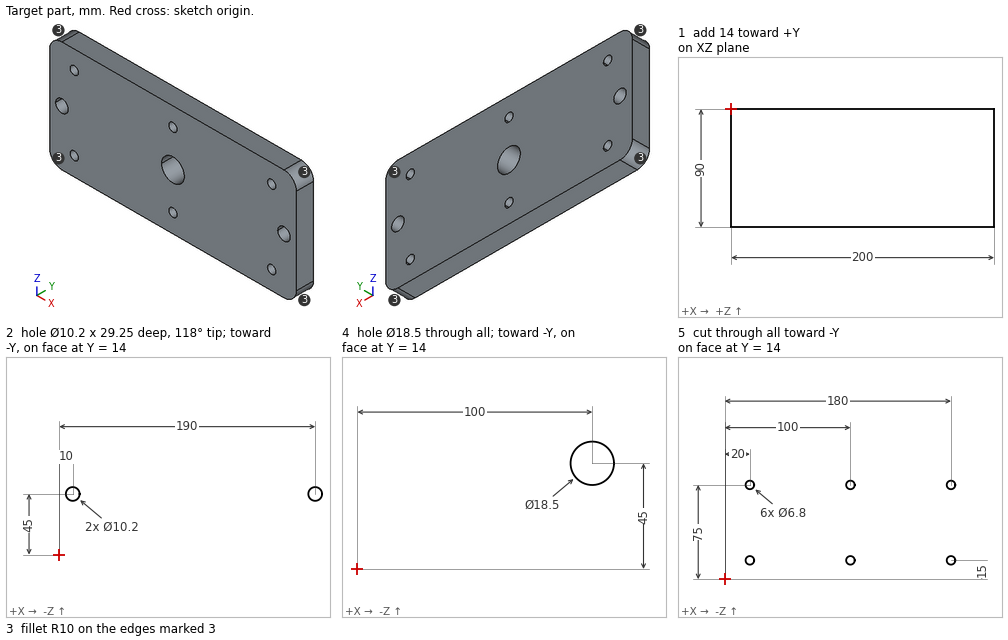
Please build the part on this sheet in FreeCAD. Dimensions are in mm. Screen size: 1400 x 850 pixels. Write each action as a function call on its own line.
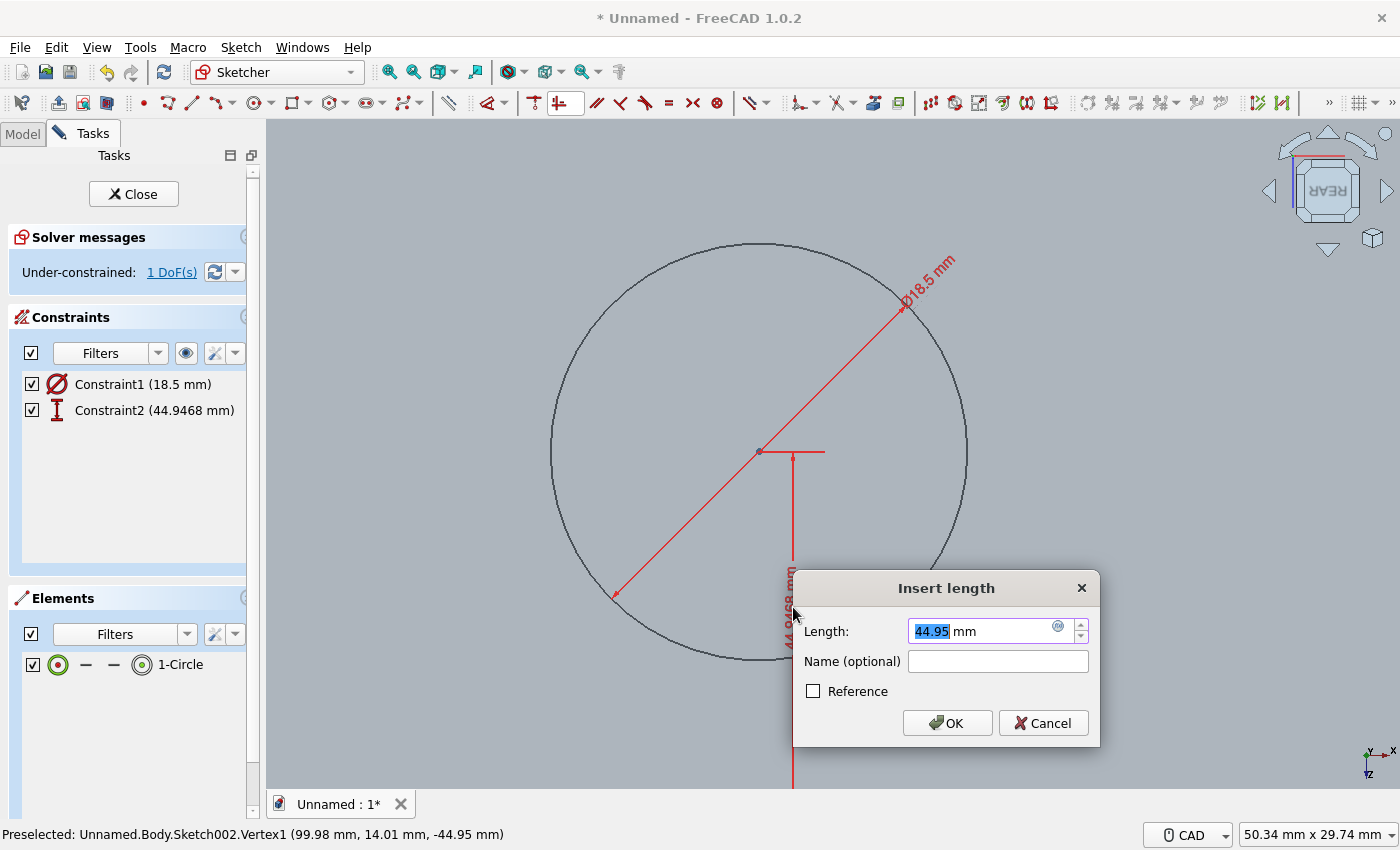
text(45)
key(Return)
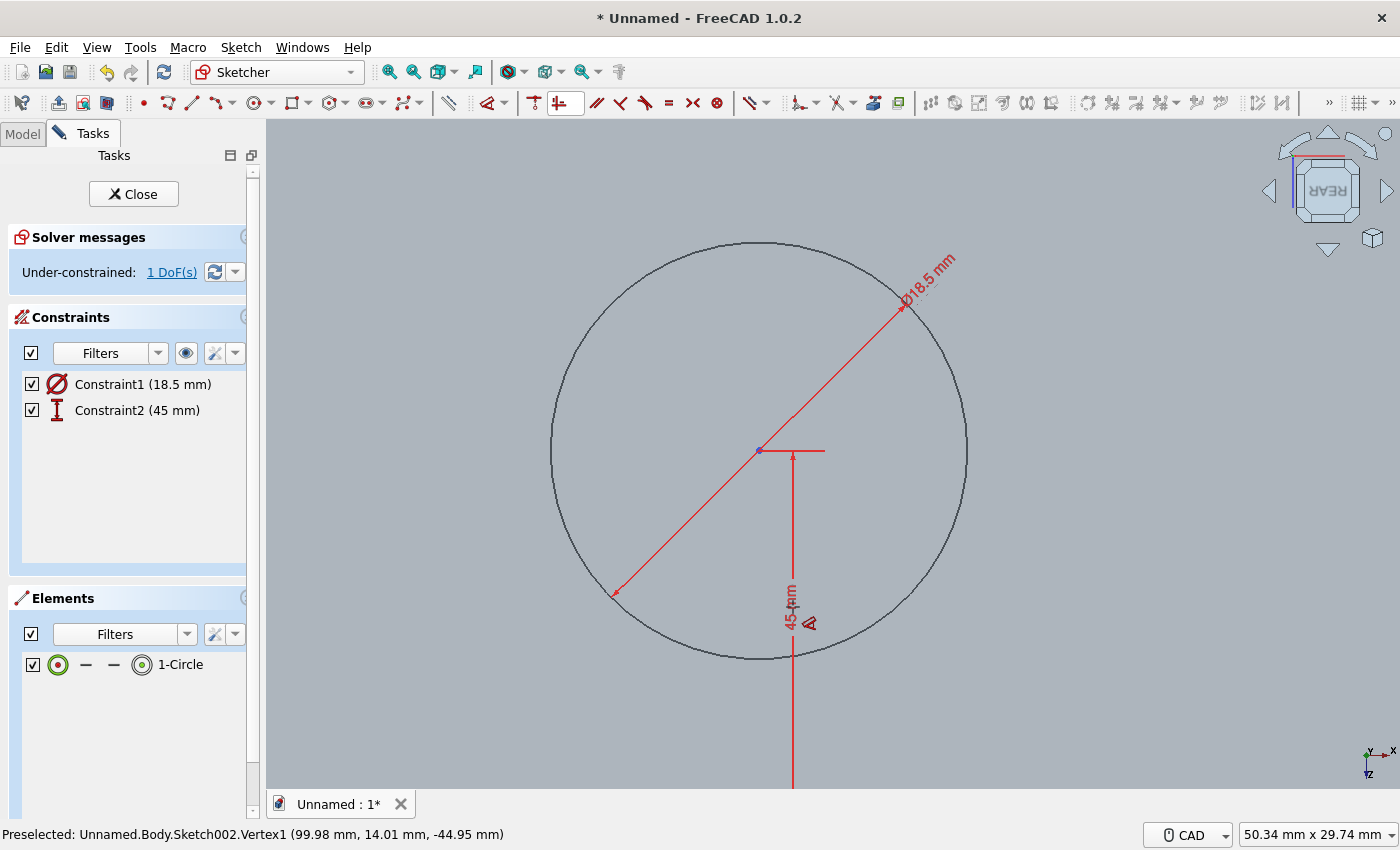
click(759, 451)
click(526, 417)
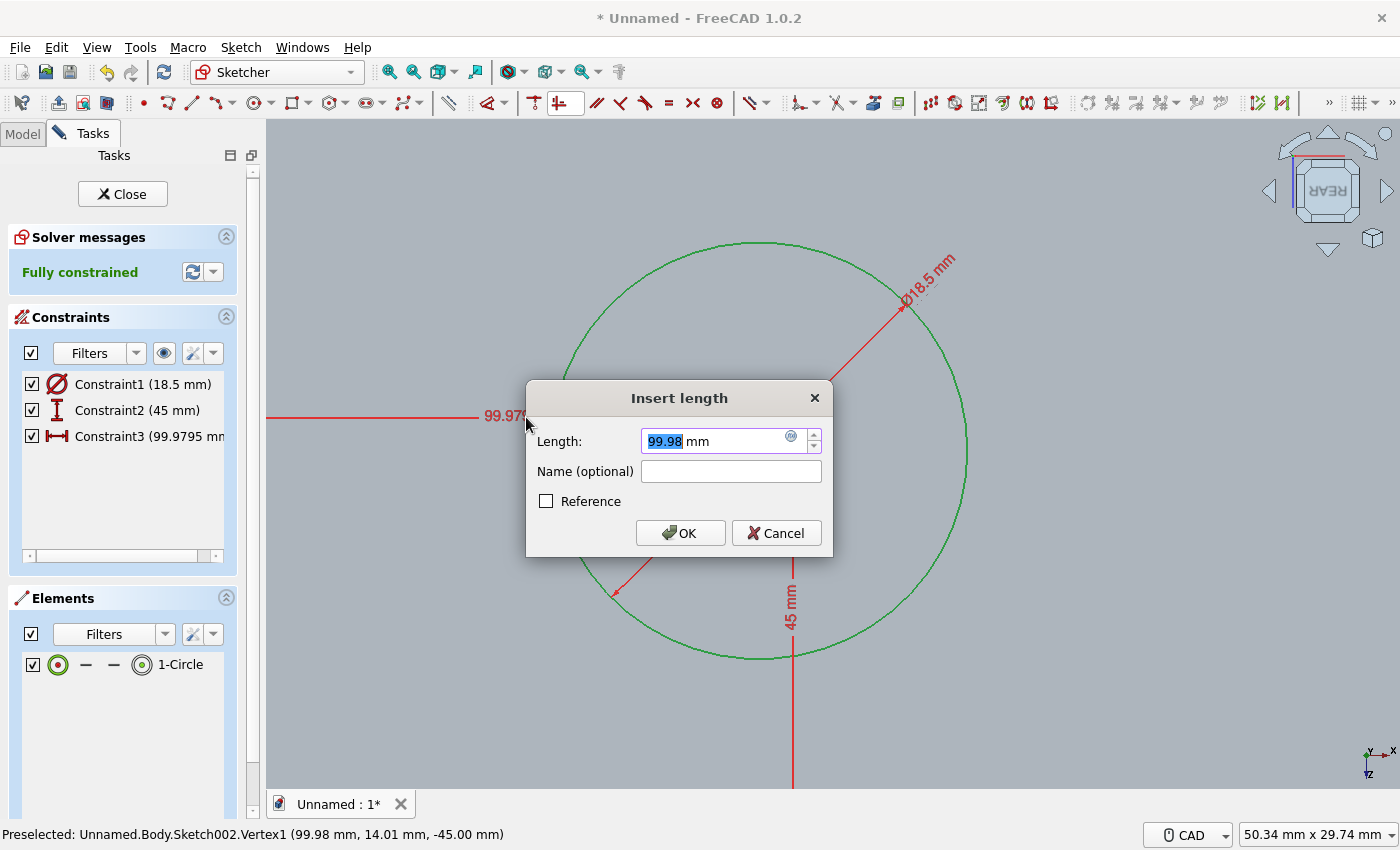
text(100)
key(Return)
key(Escape)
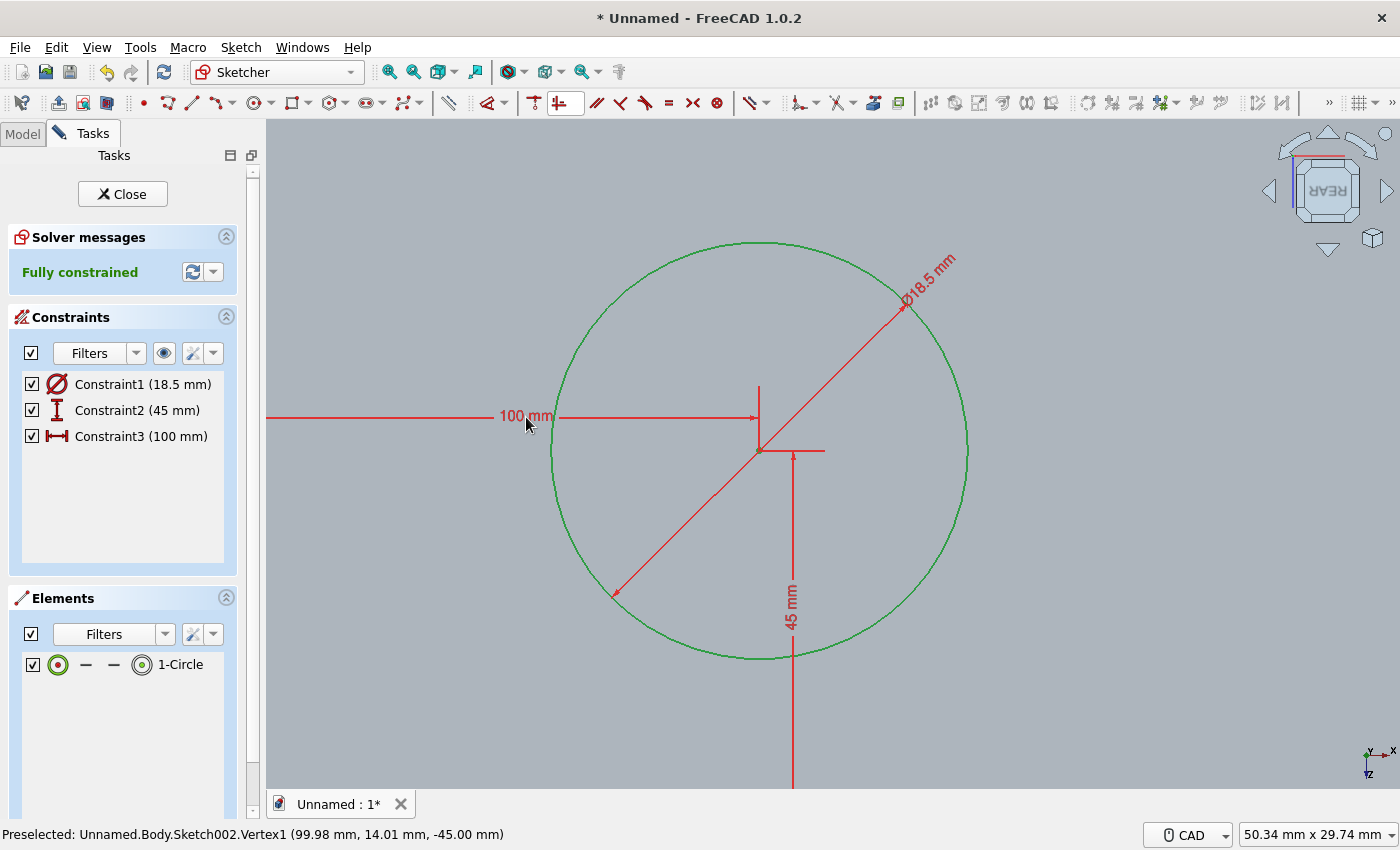
click(123, 194)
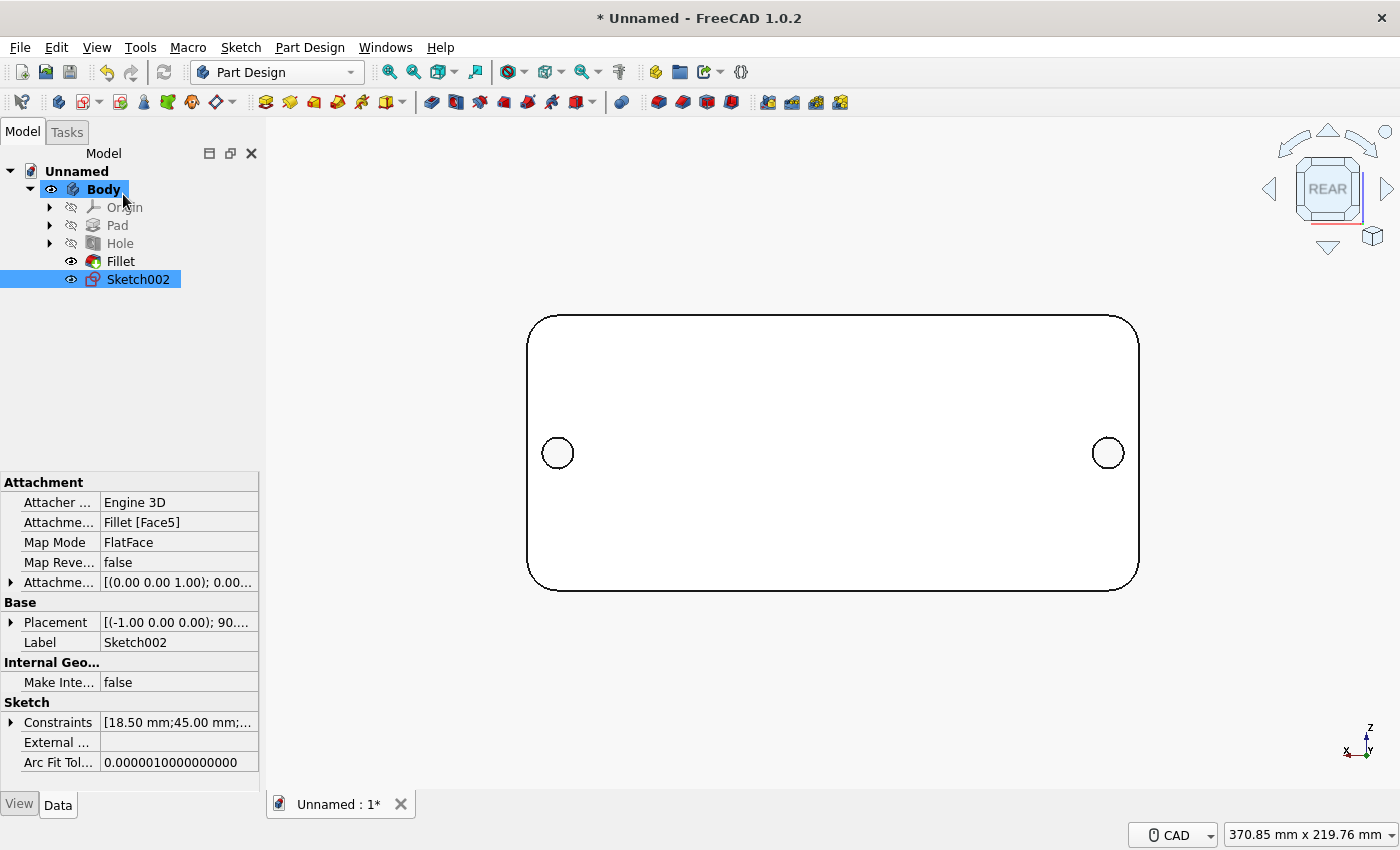
click(456, 102)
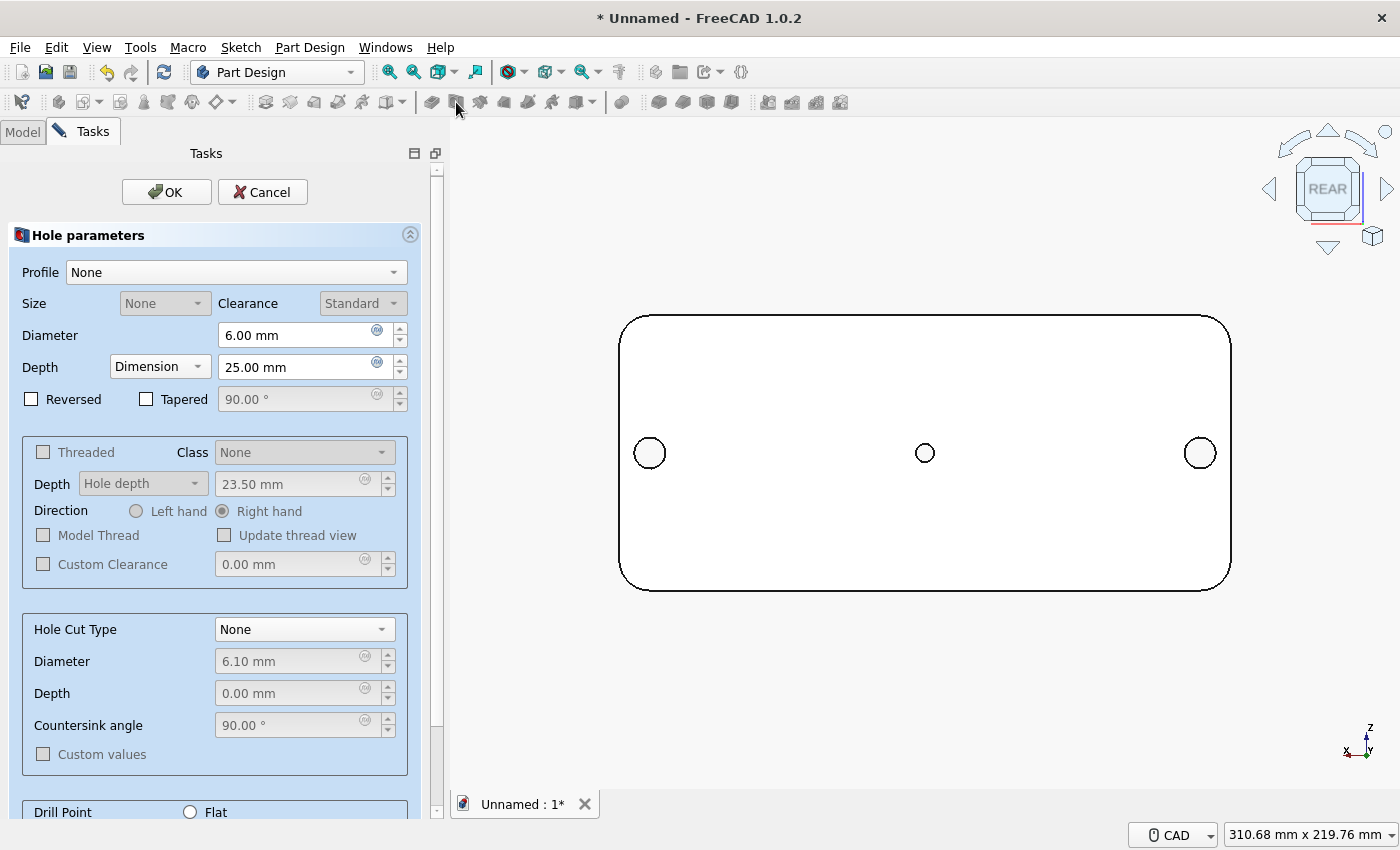
triple_click(305, 335)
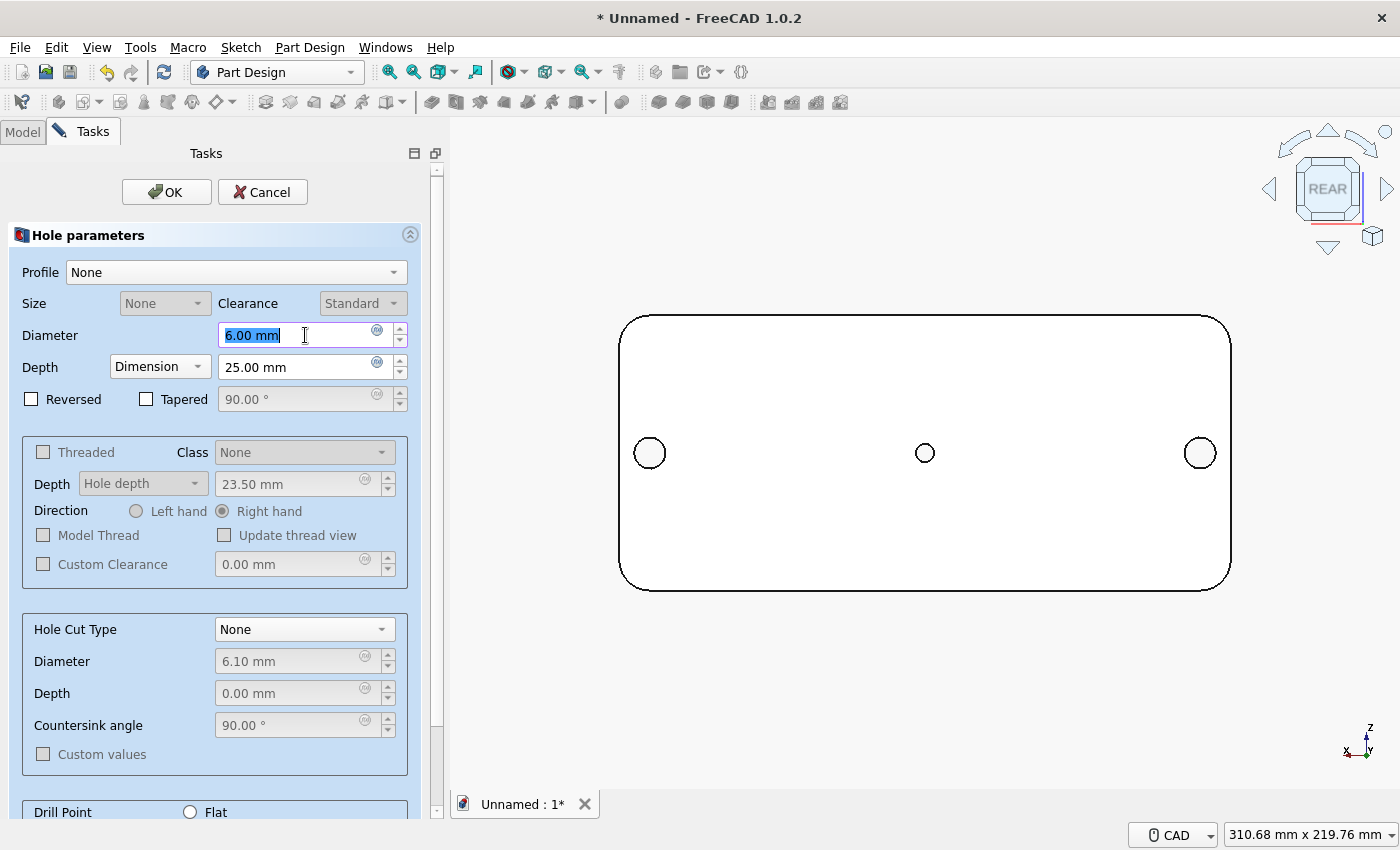
text(18.5)
key(Tab)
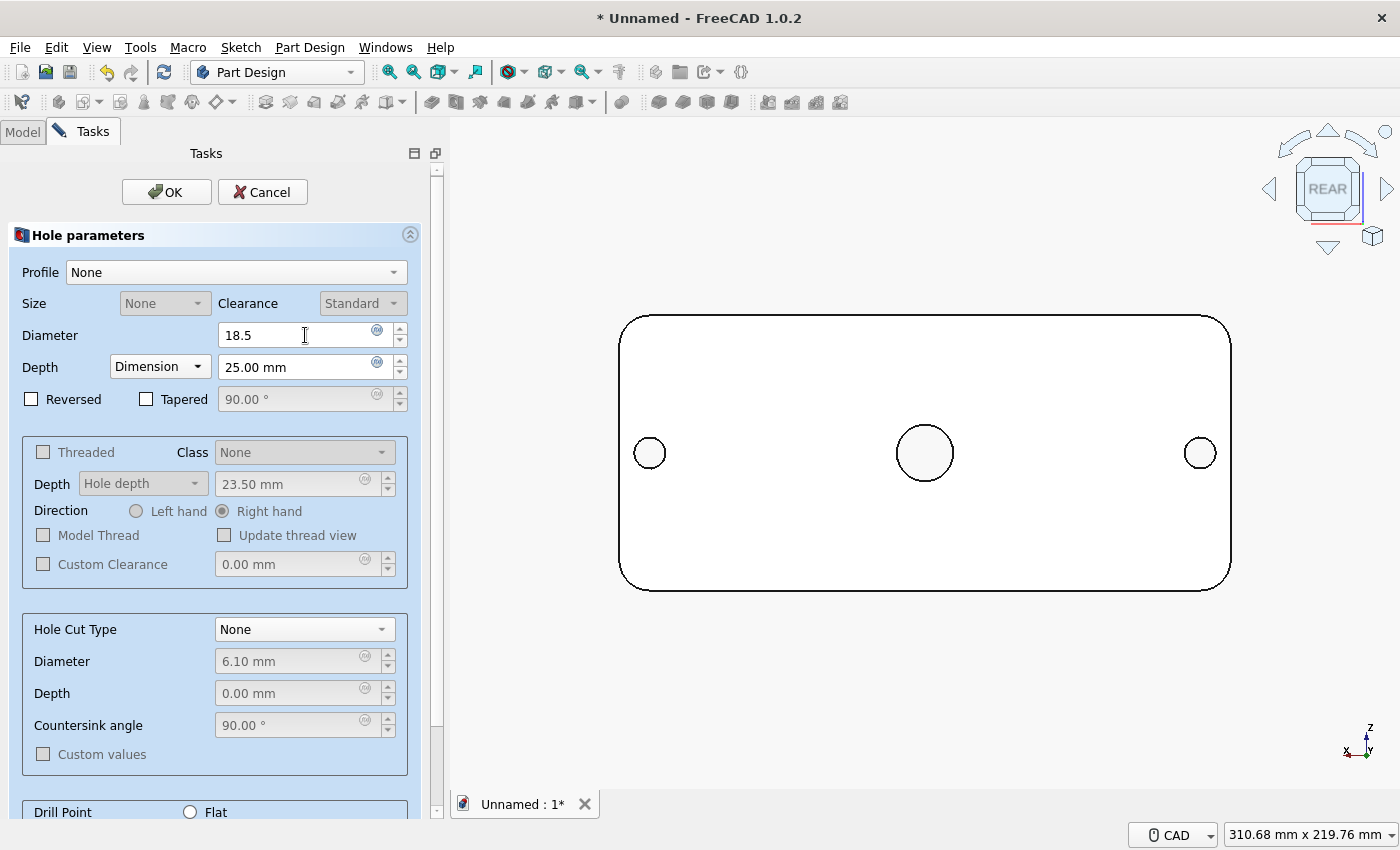
click(161, 366)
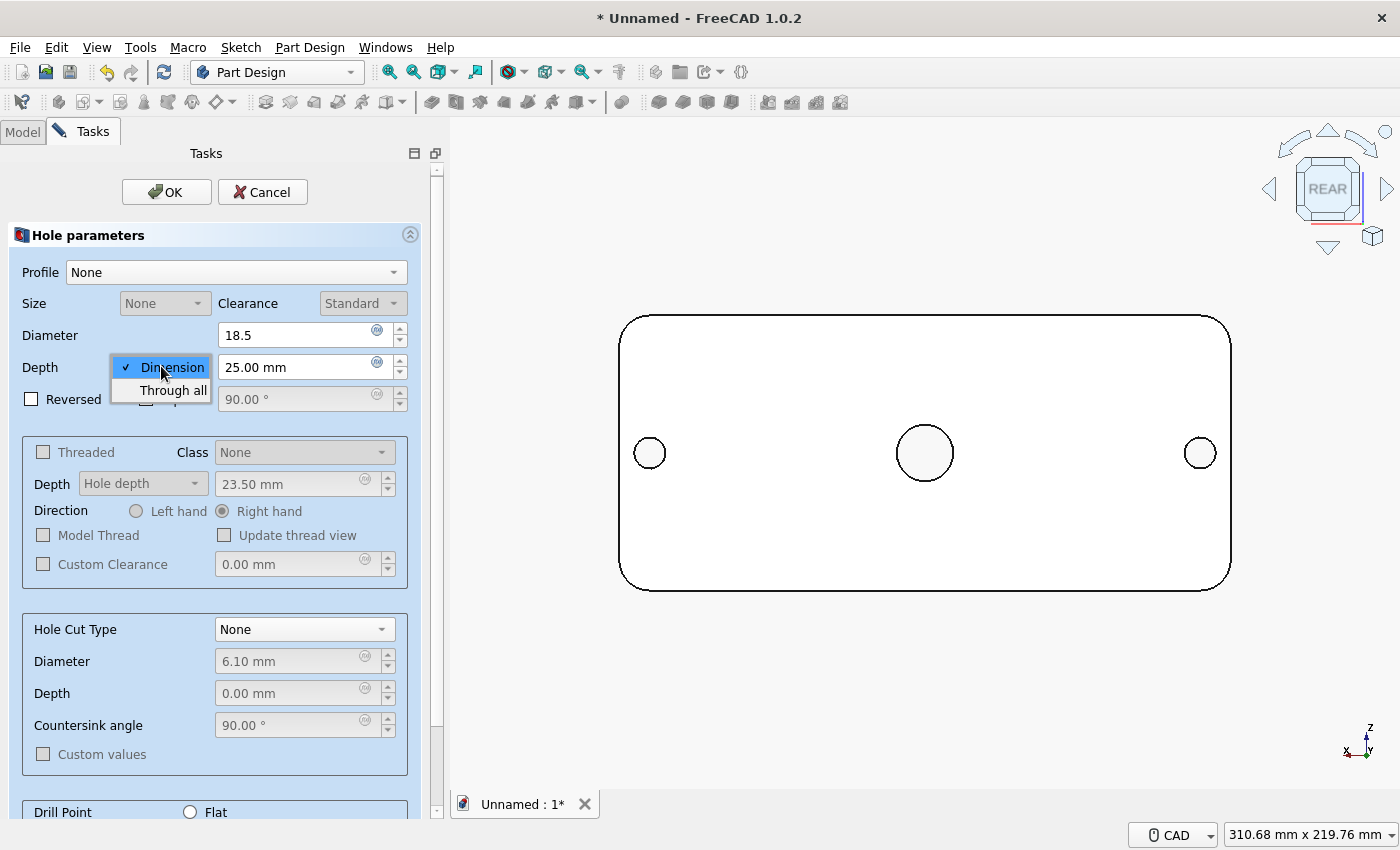
click(160, 390)